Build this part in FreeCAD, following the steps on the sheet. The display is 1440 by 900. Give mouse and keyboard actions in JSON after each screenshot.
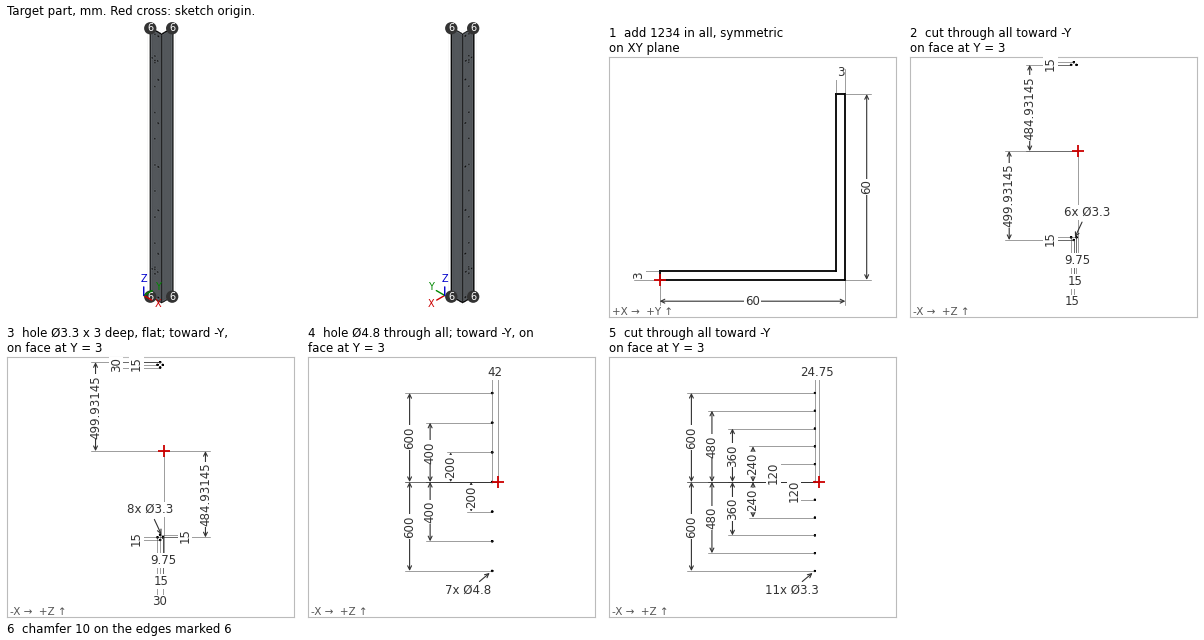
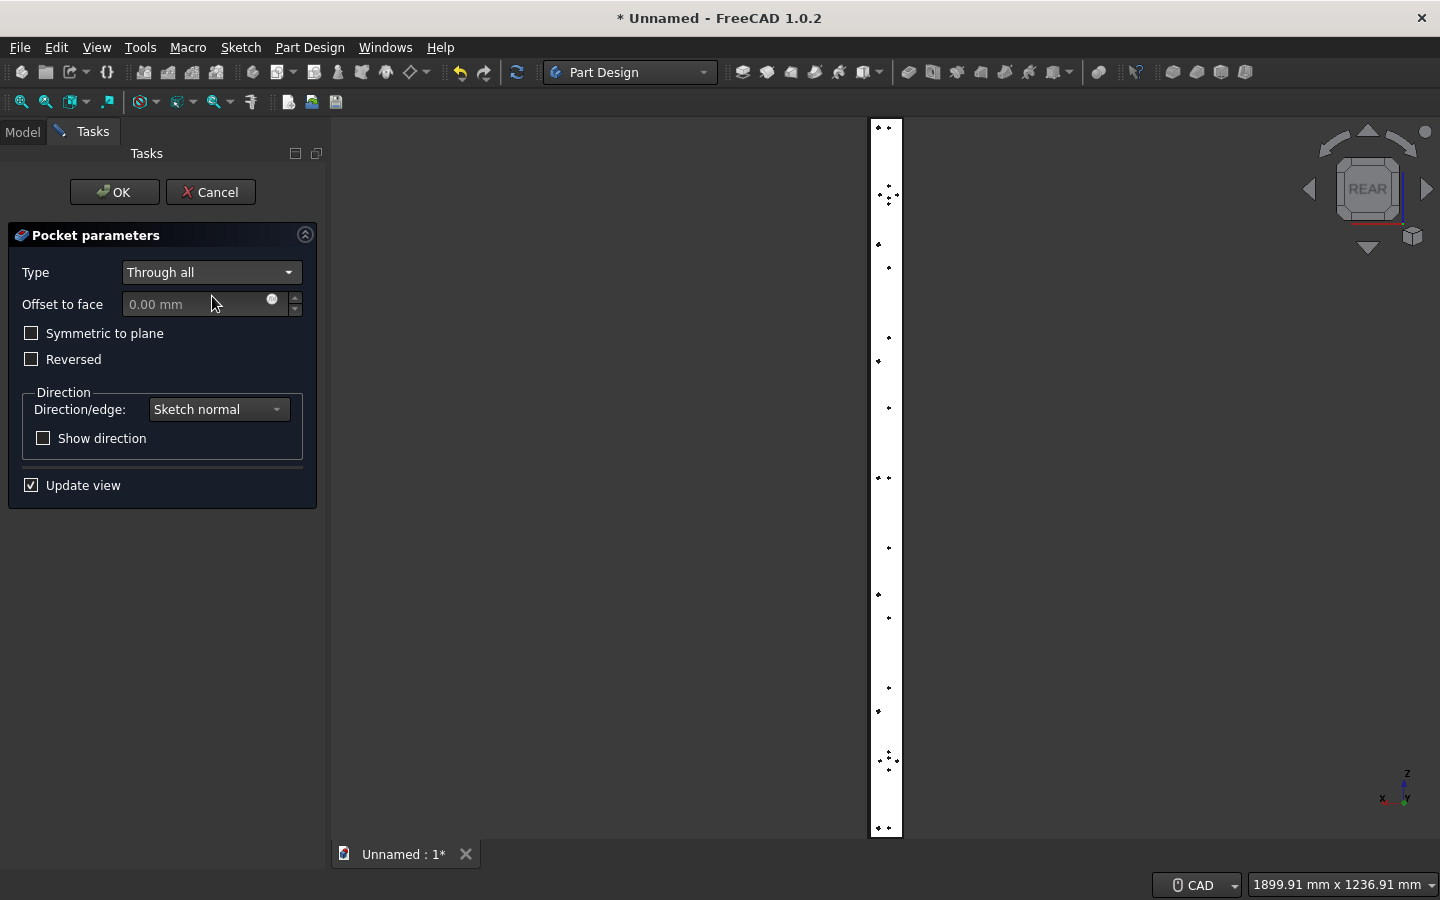
{"action": "left_click", "coordinate": [115, 192]}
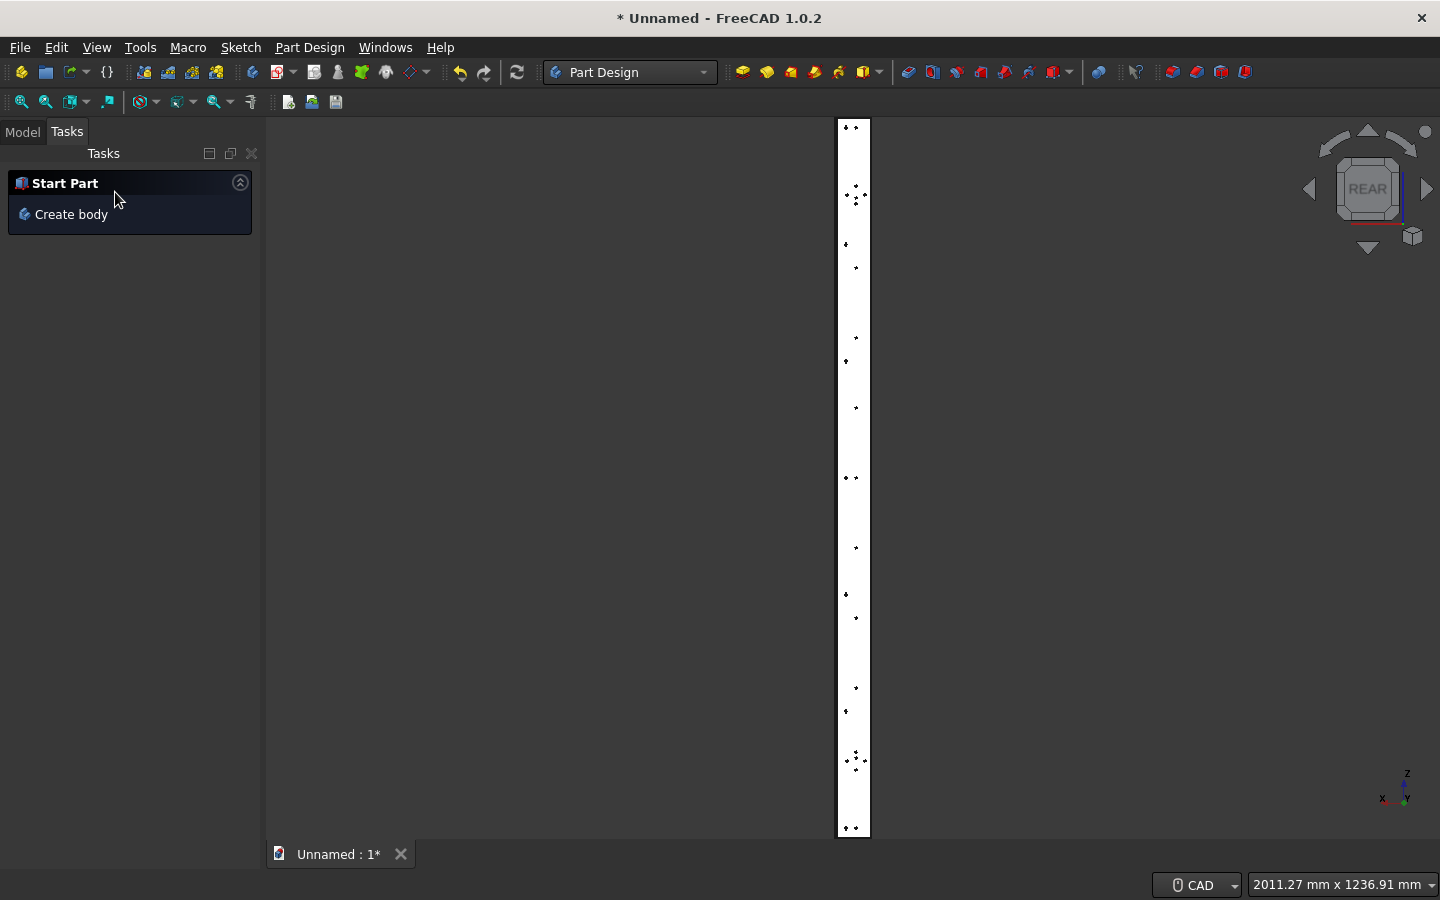
{"action": "key", "text": "0"}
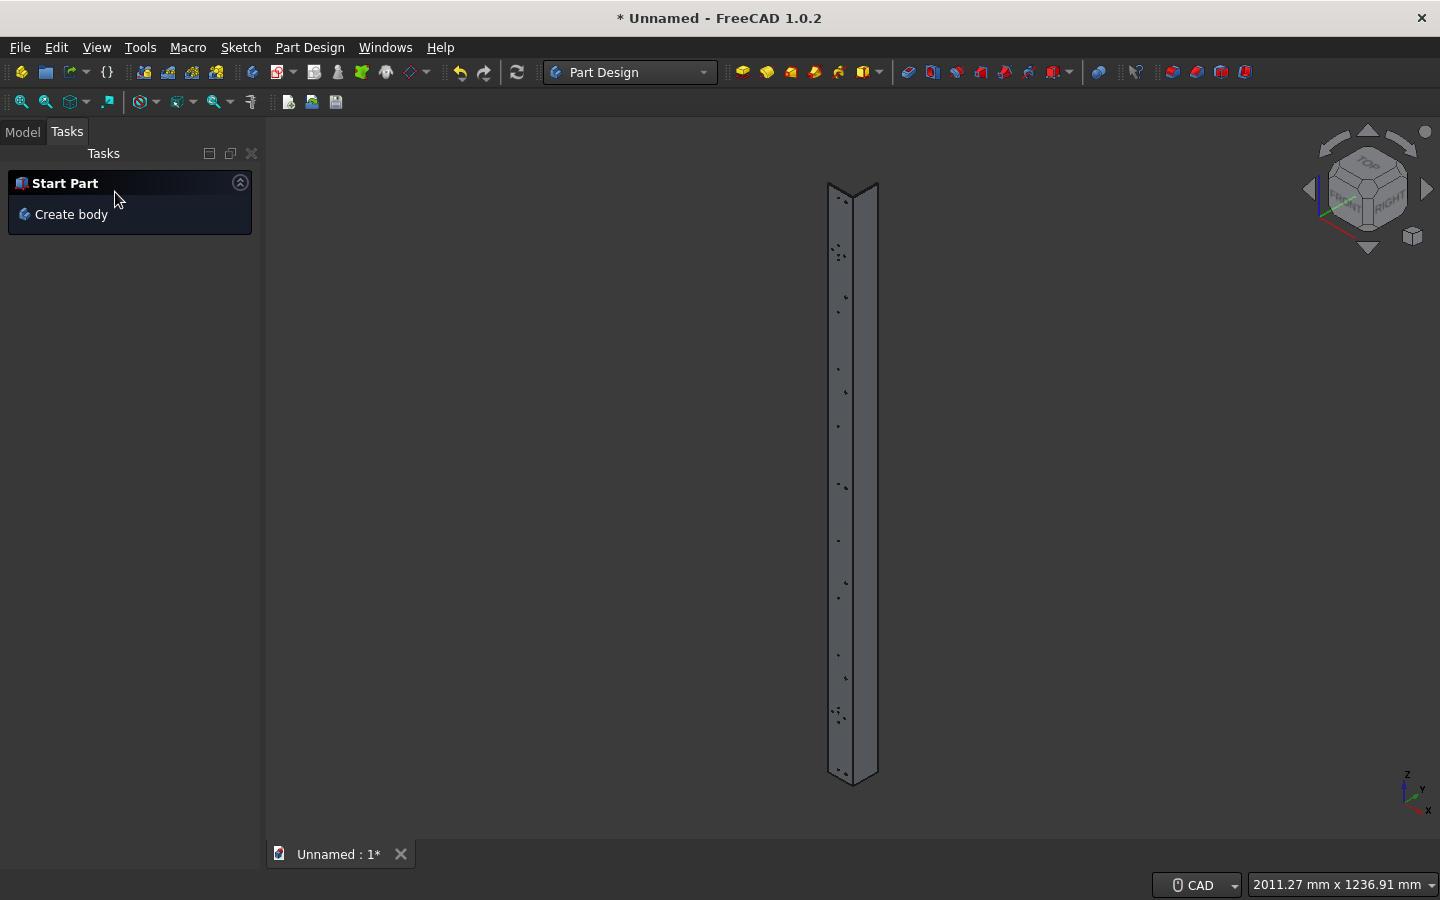
{"action": "scroll", "coordinate": [877, 183], "scroll_direction": "up", "scroll_amount": 15}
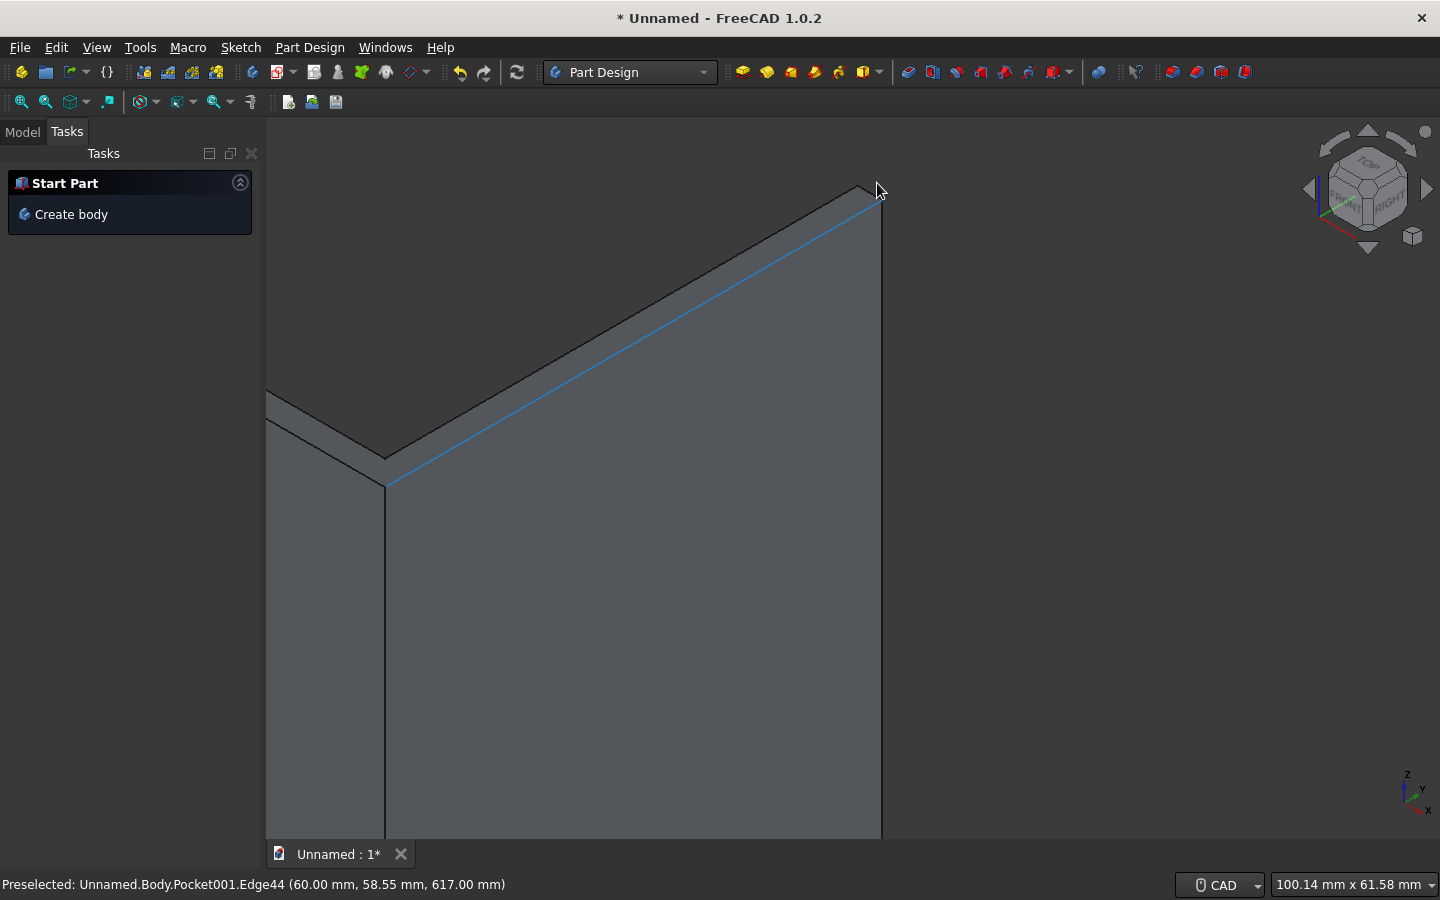
{"action": "left_click", "coordinate": [22, 102]}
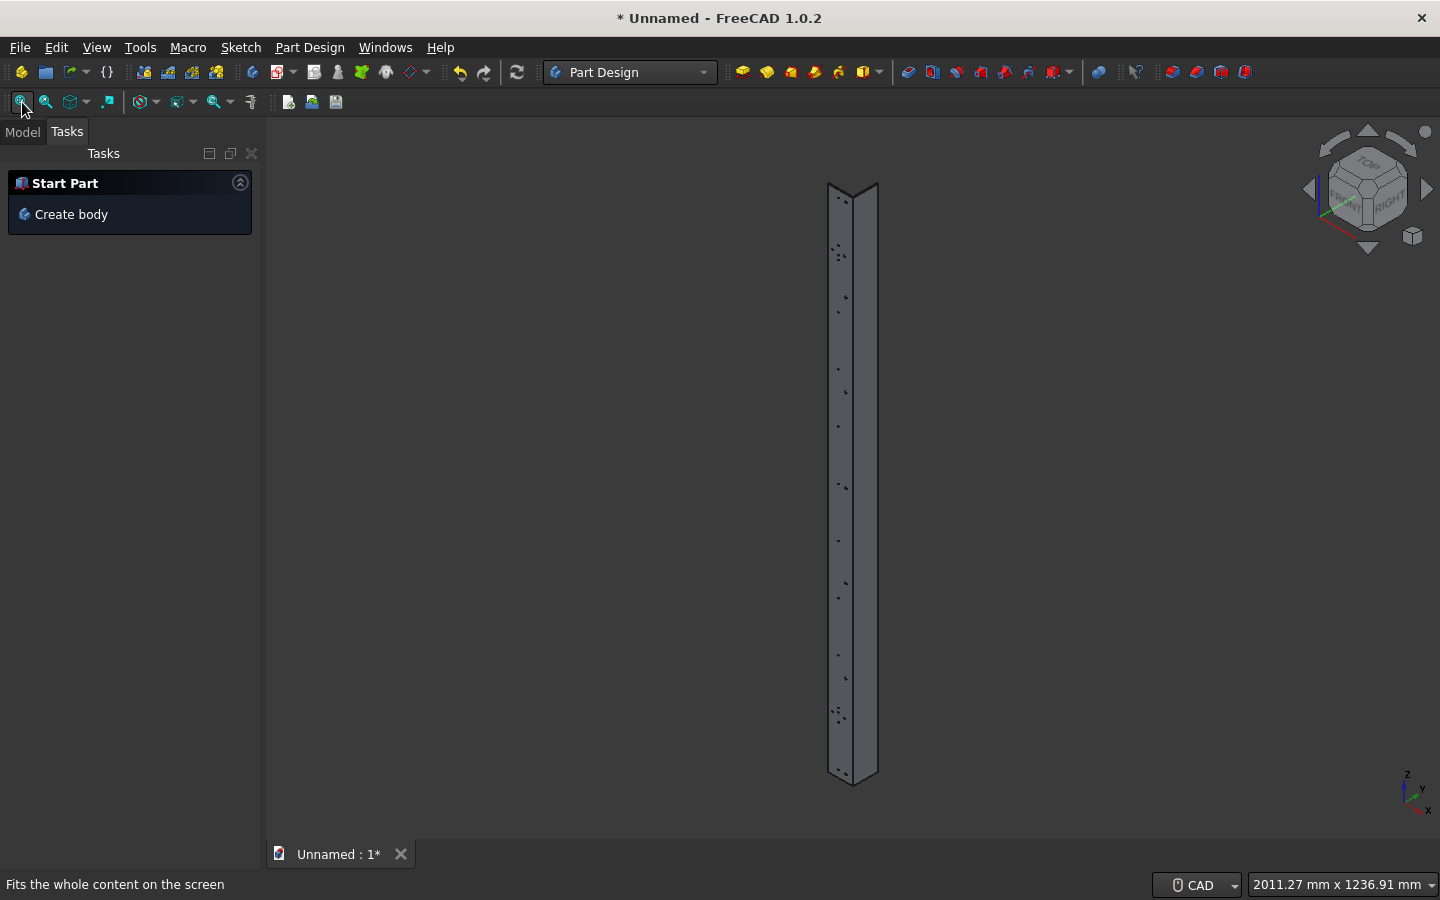
{"action": "key", "text": "2"}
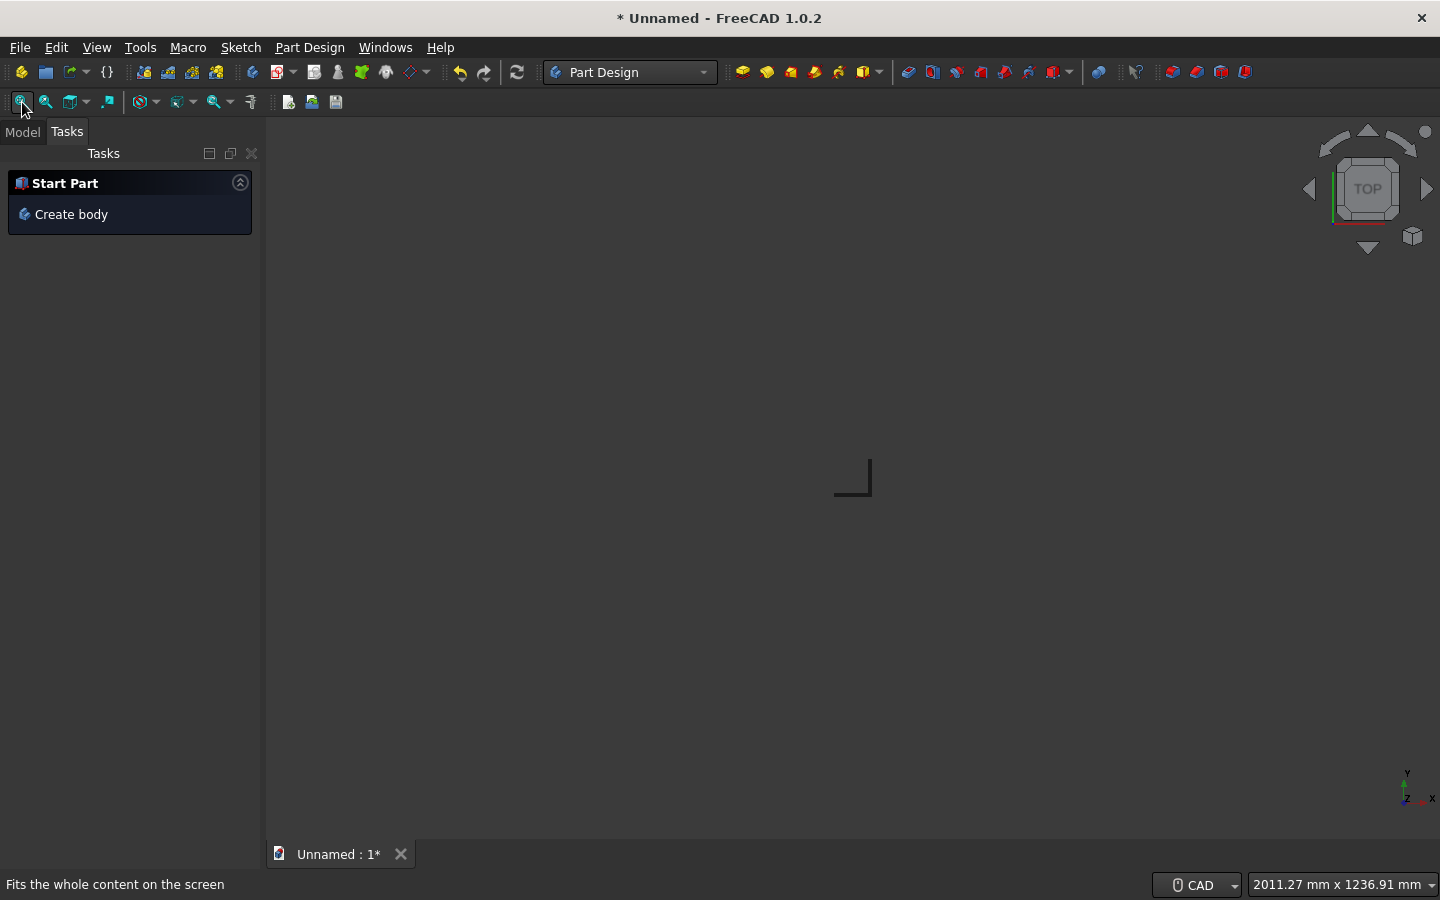
{"action": "left_click", "coordinate": [22, 102]}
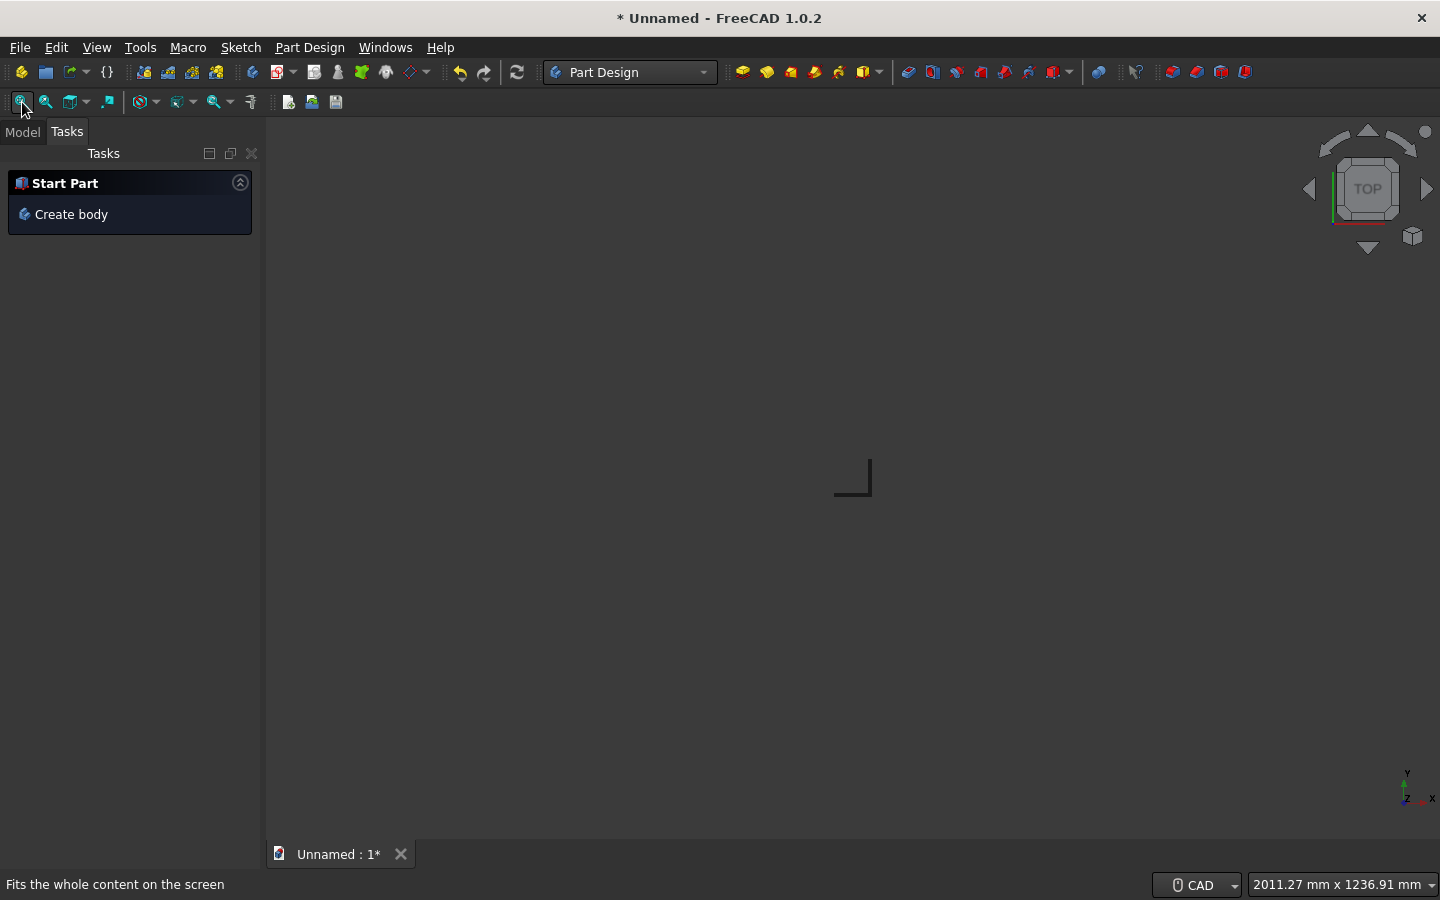
{"action": "scroll", "coordinate": [870, 459], "scroll_direction": "up", "scroll_amount": 15}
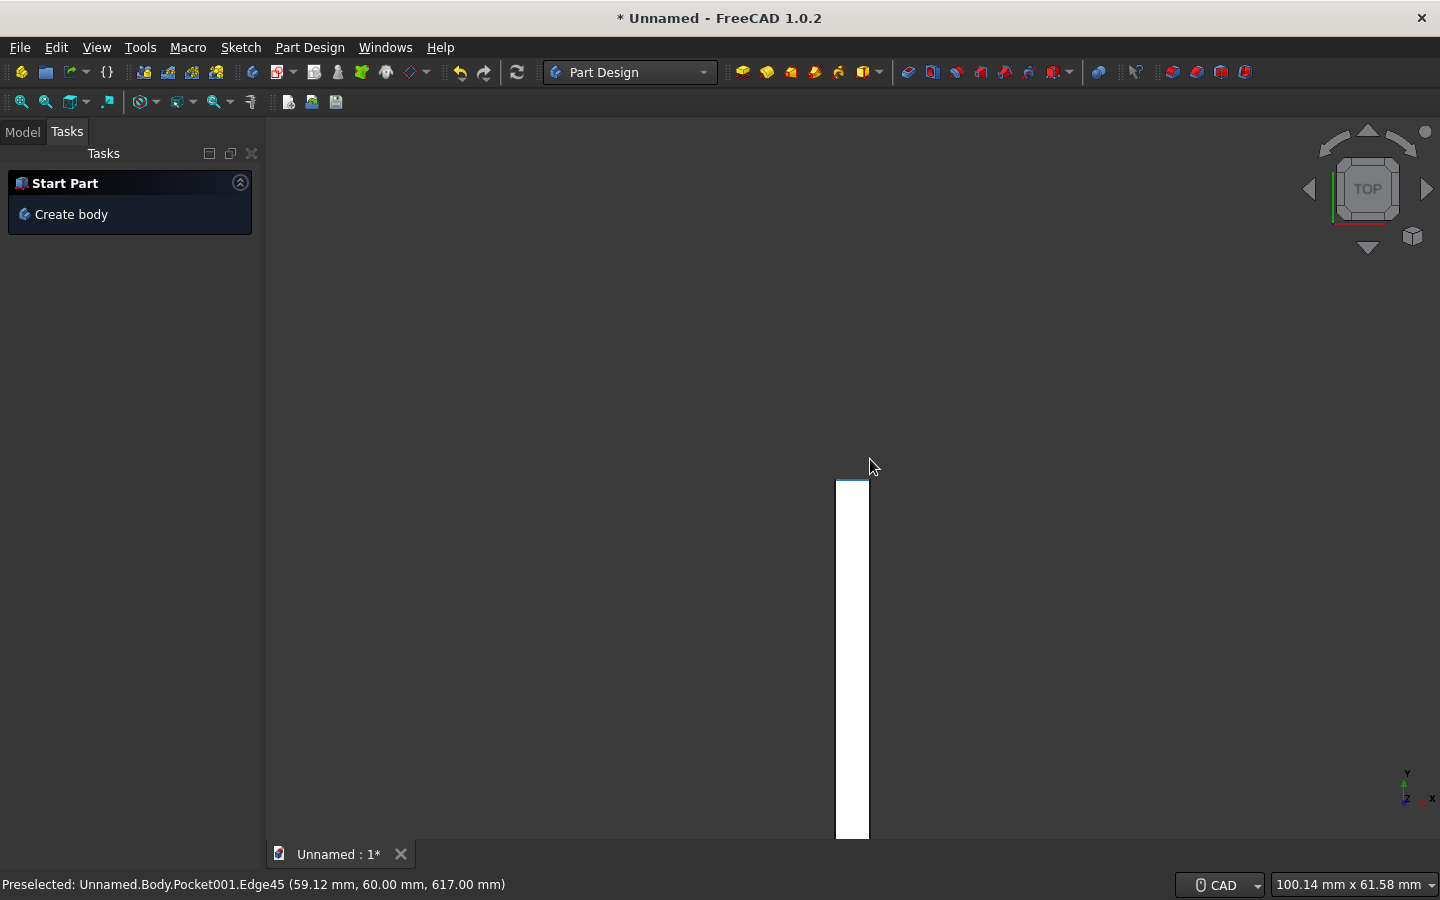
{"action": "left_click", "coordinate": [853, 479]}